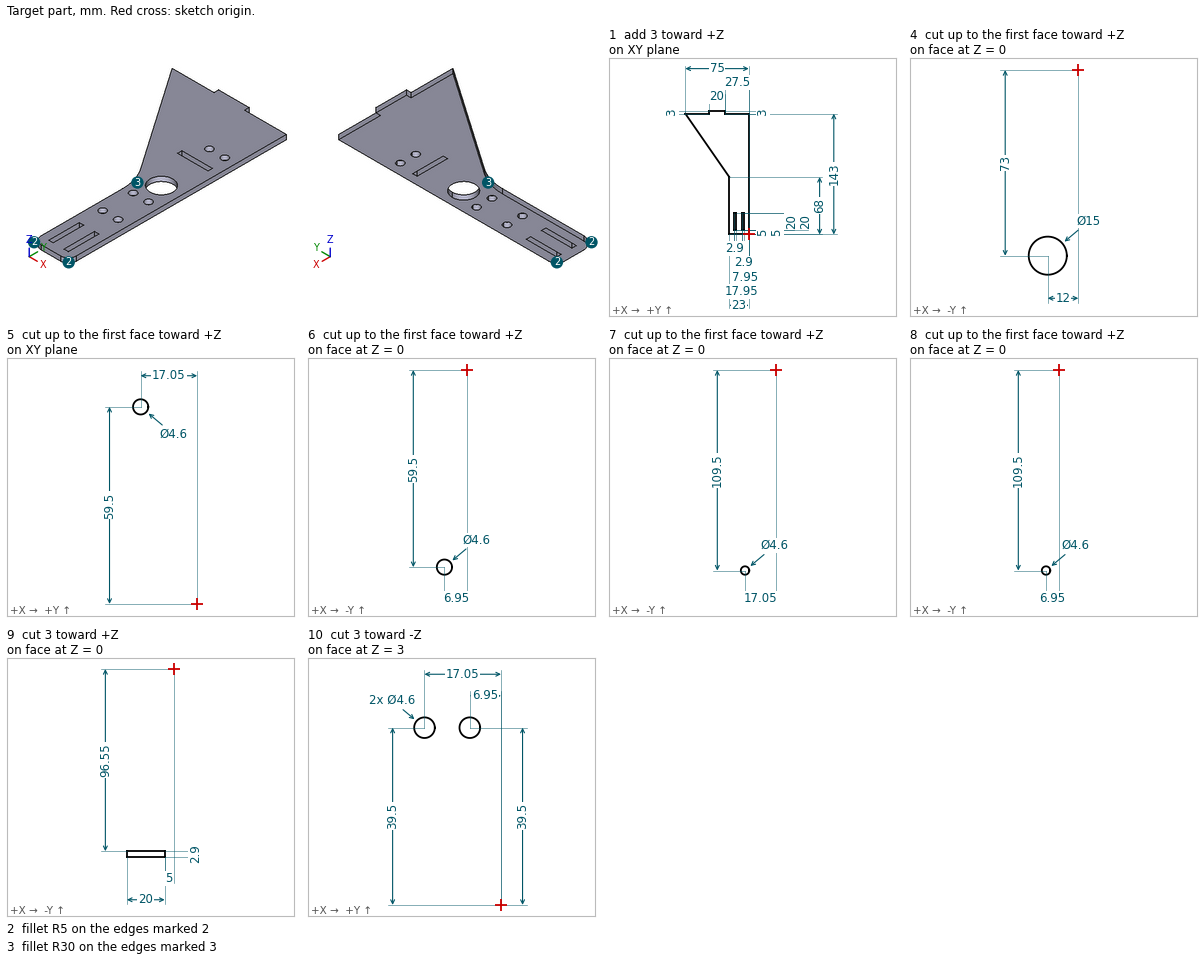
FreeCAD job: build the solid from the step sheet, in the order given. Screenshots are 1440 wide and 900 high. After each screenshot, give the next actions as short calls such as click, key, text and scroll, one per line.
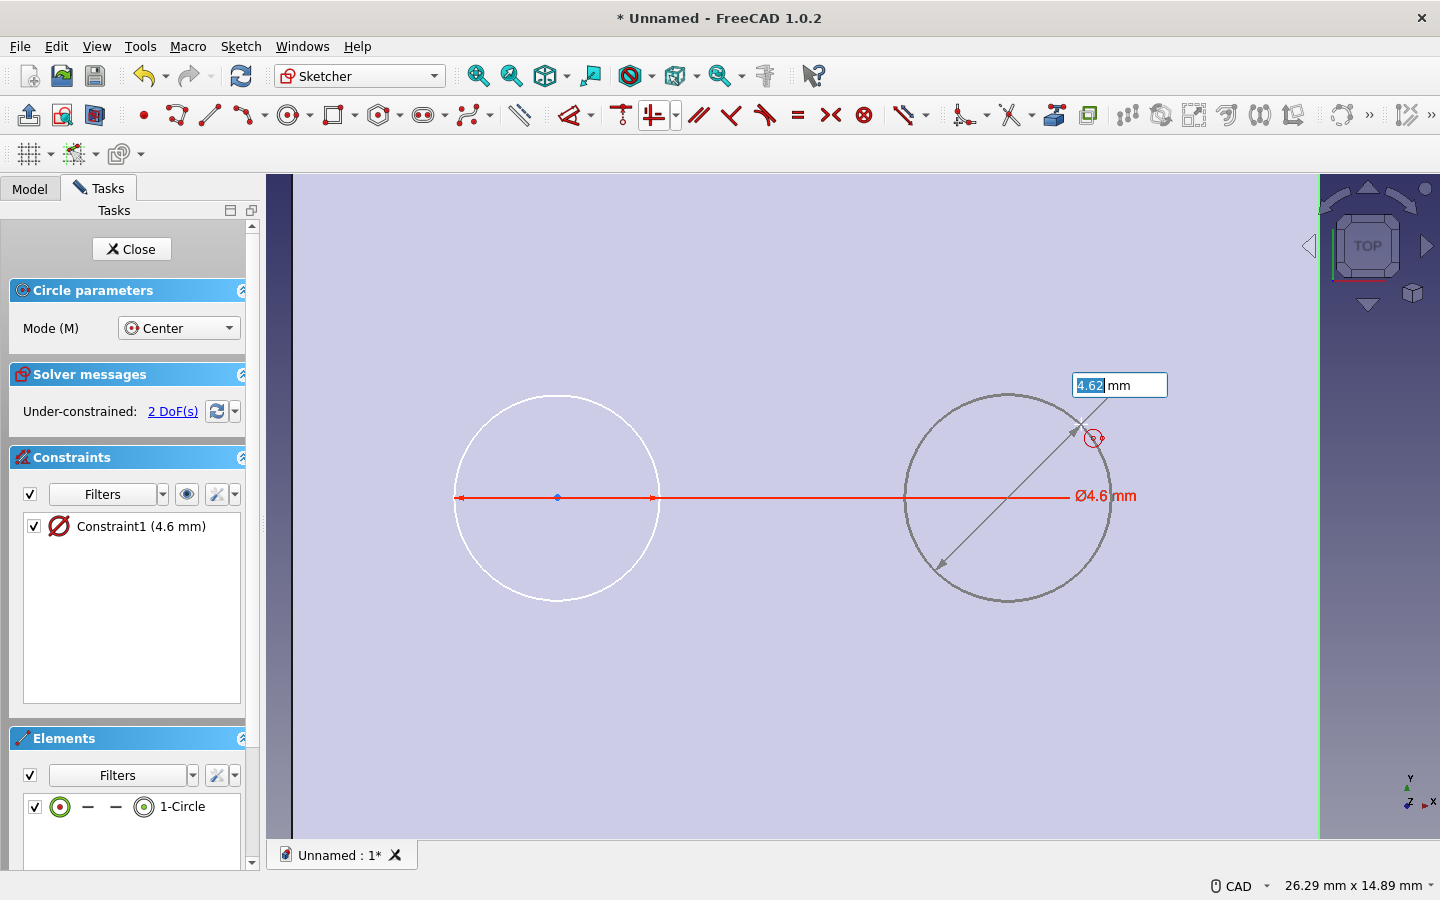
text(4.6)
key(Return)
key(Escape)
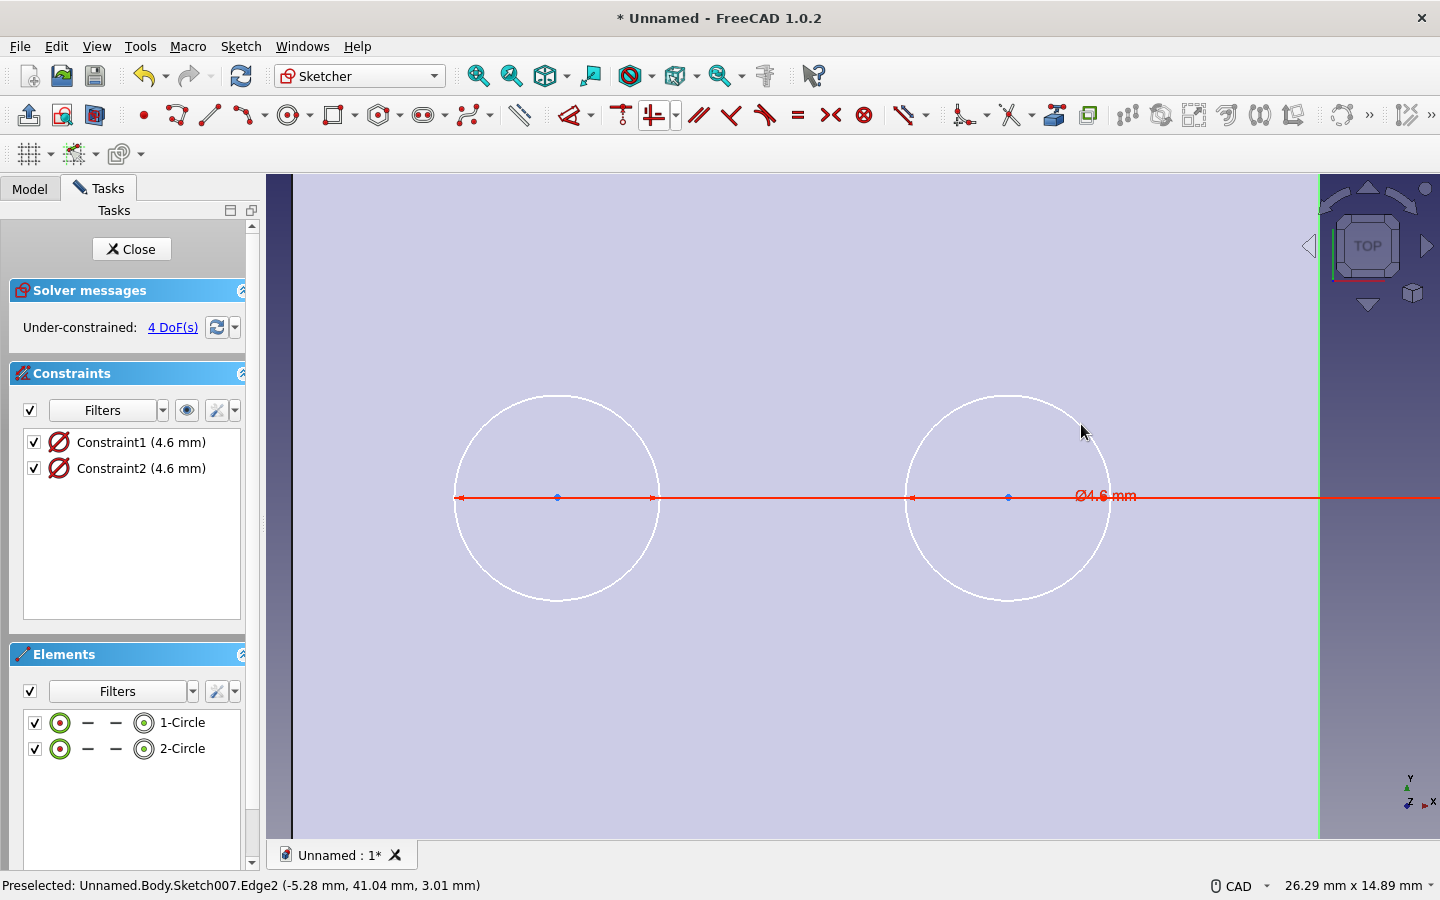
key(d)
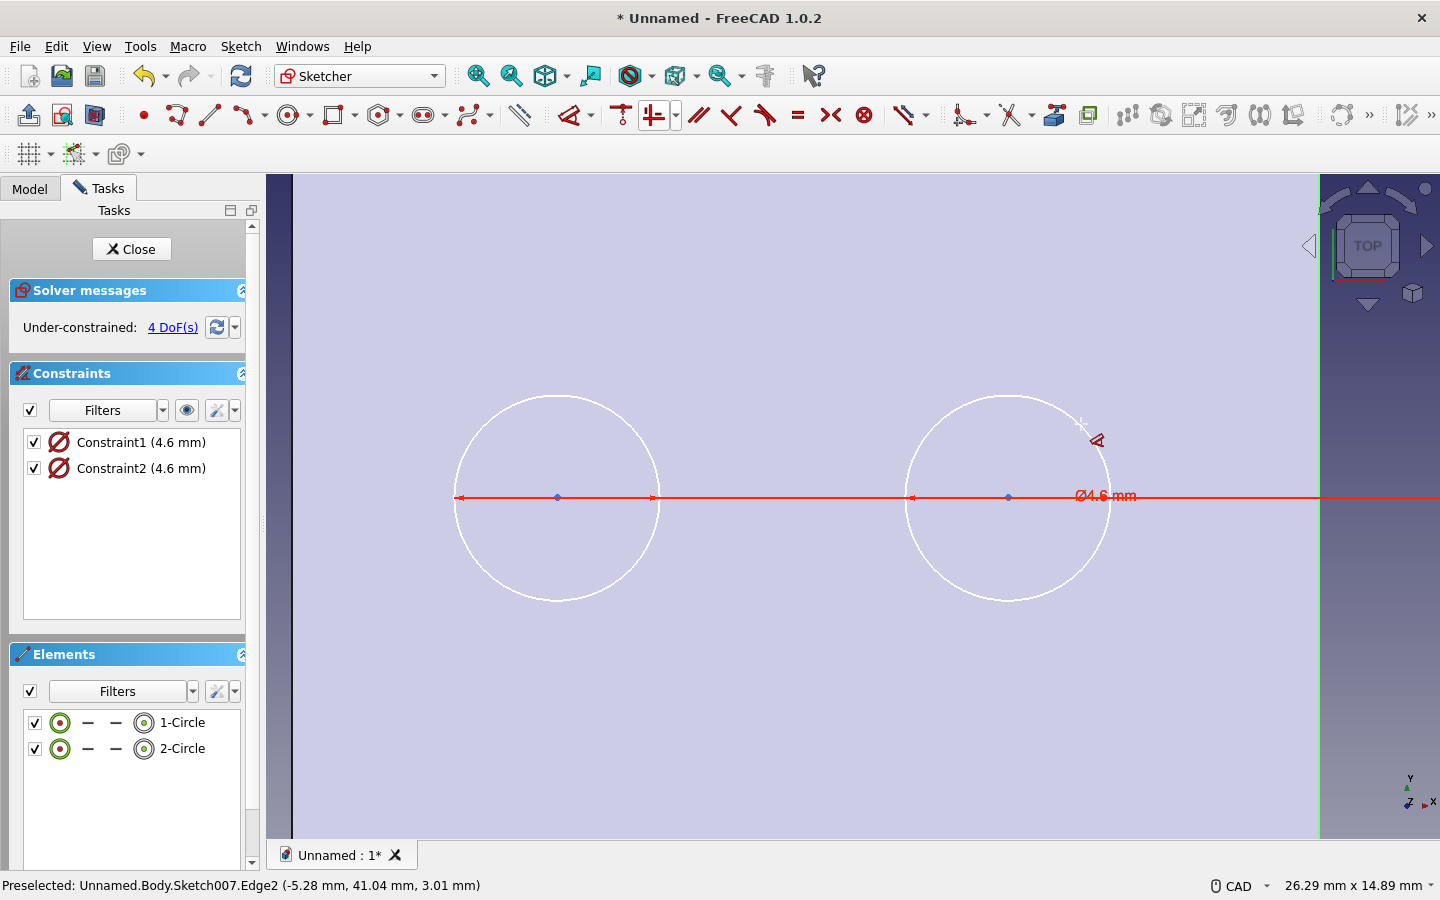
click(557, 498)
click(523, 655)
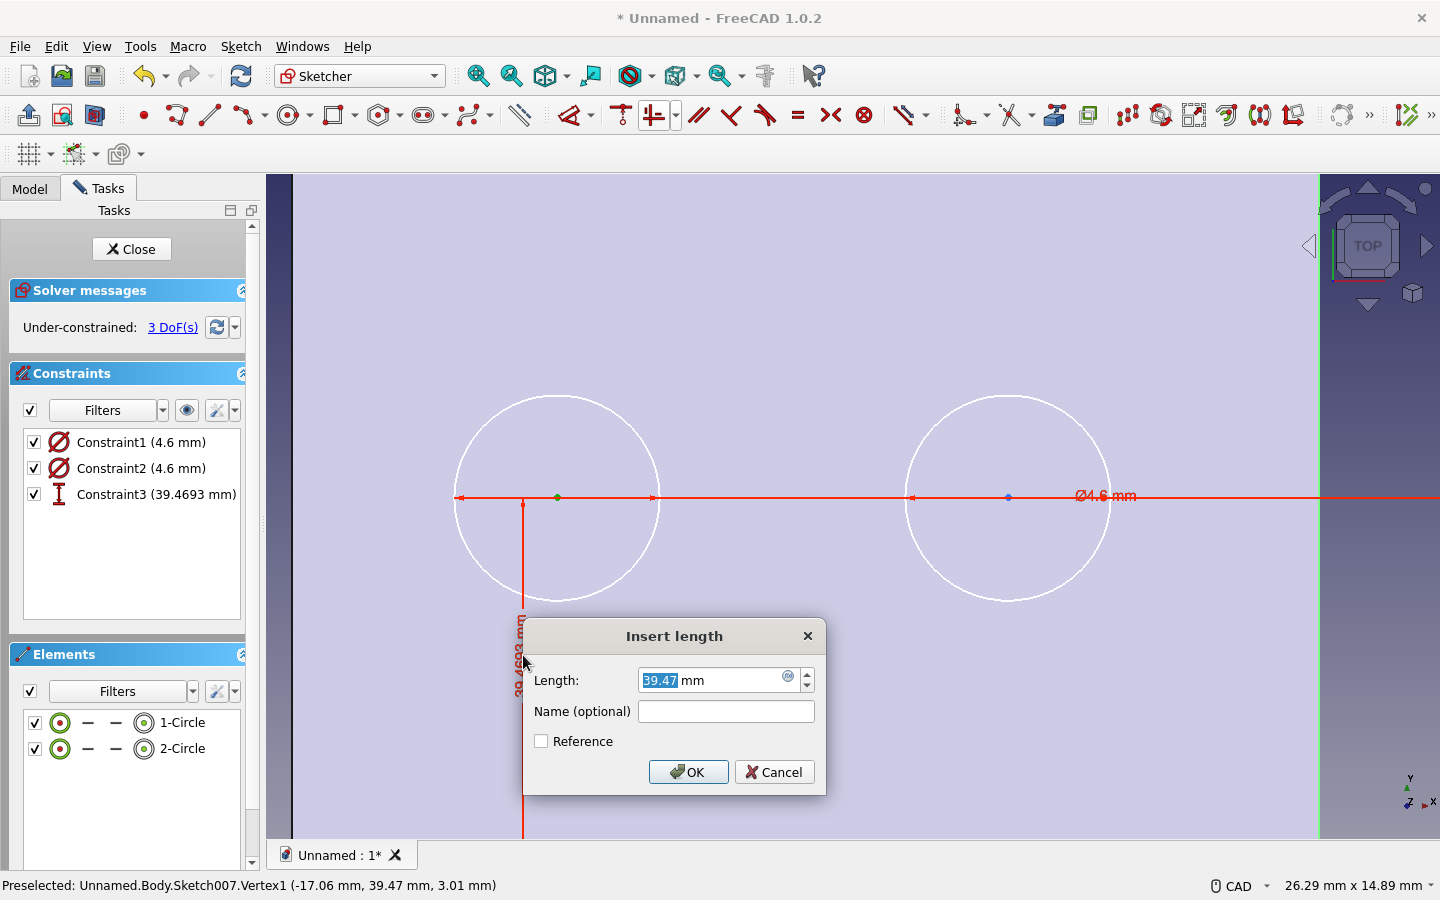
text(39.5)
key(Return)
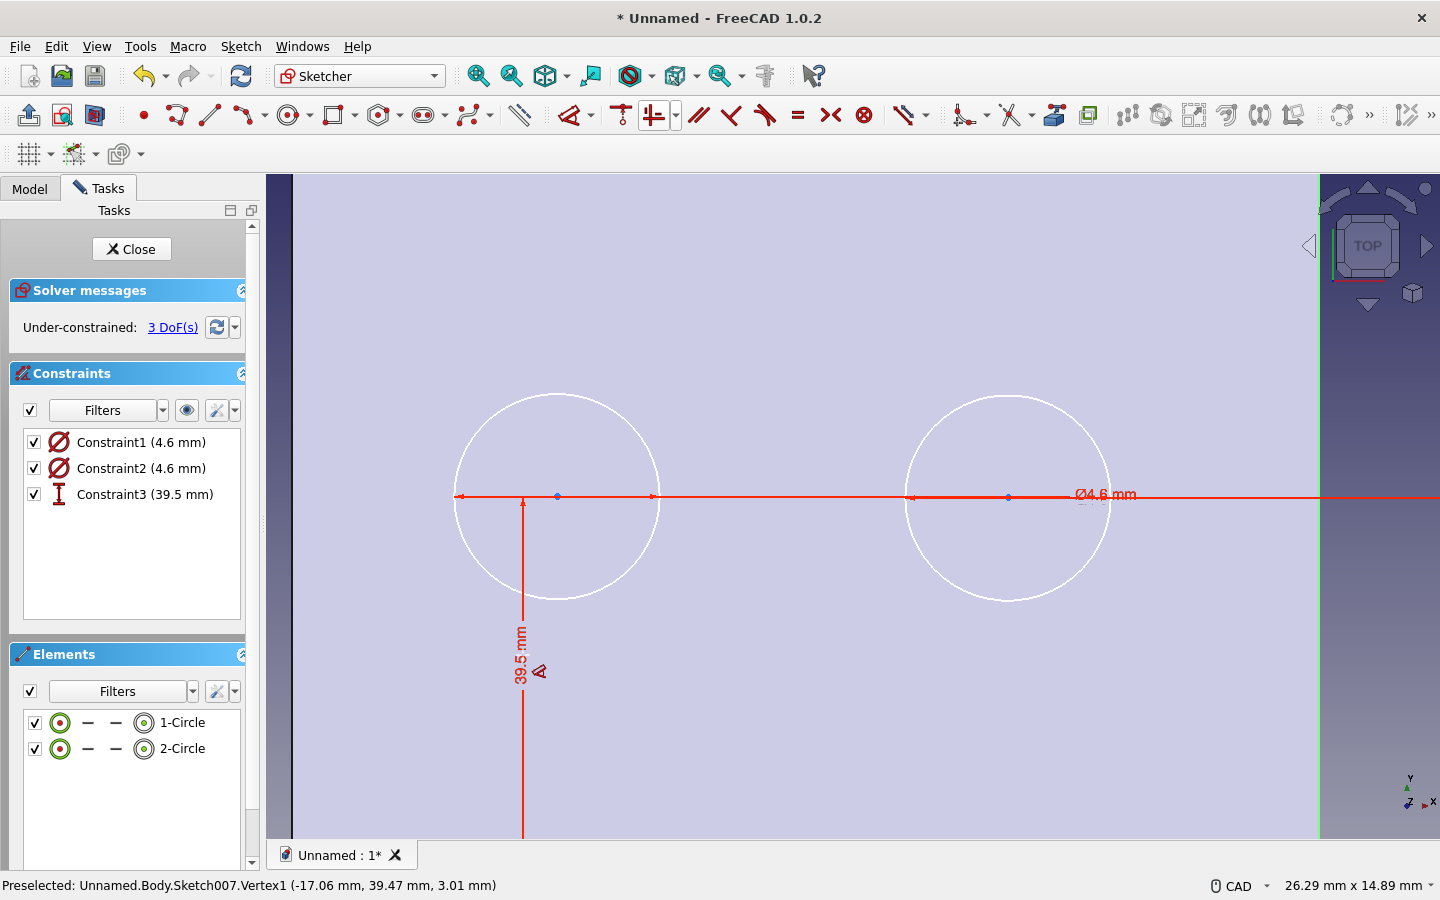
click(1008, 498)
click(1142, 464)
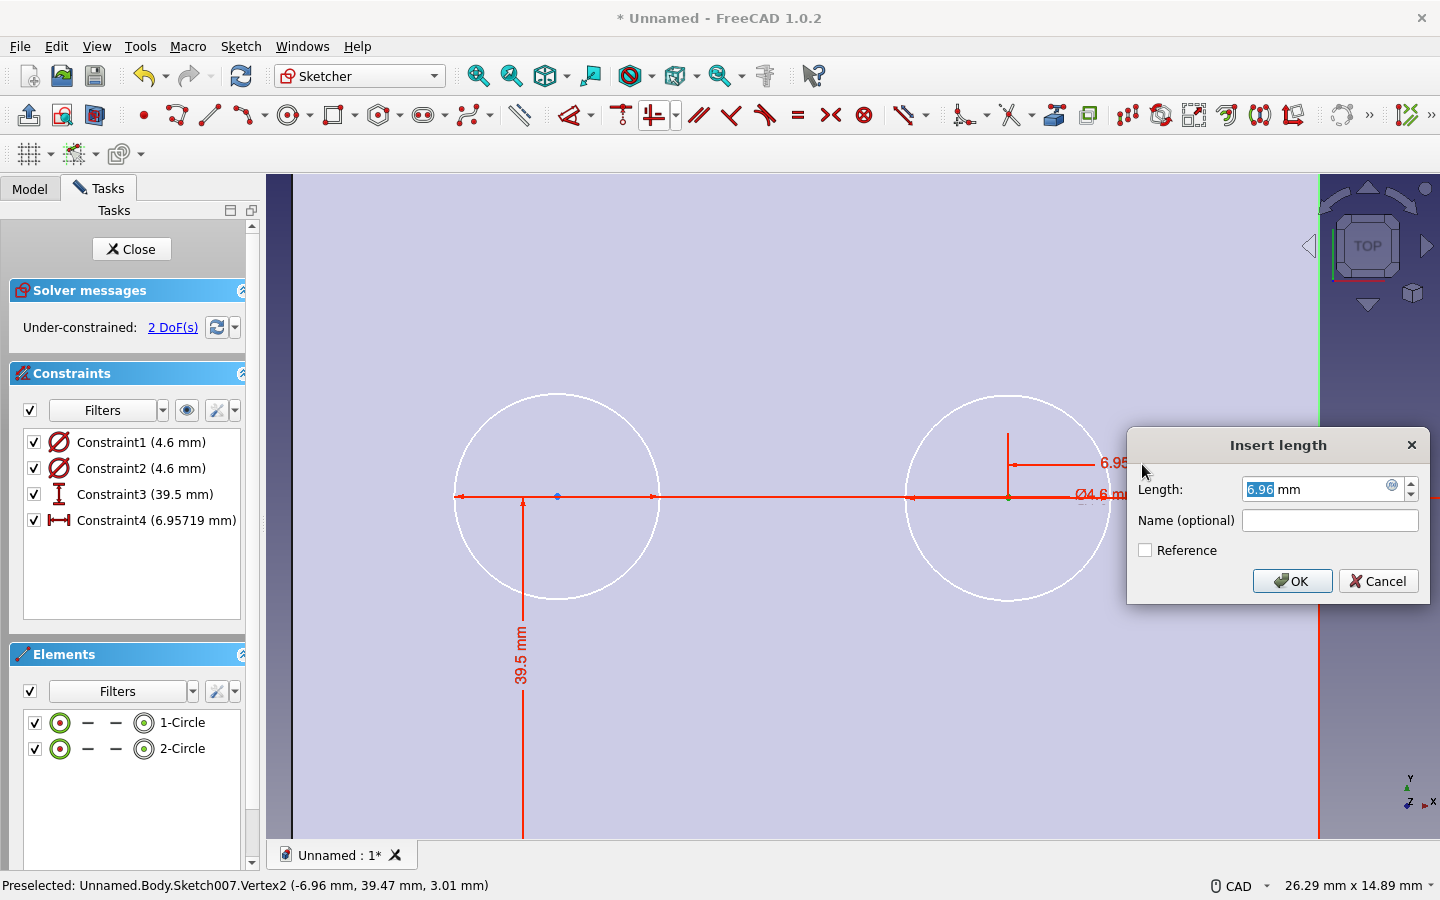
text(6.95)
key(Return)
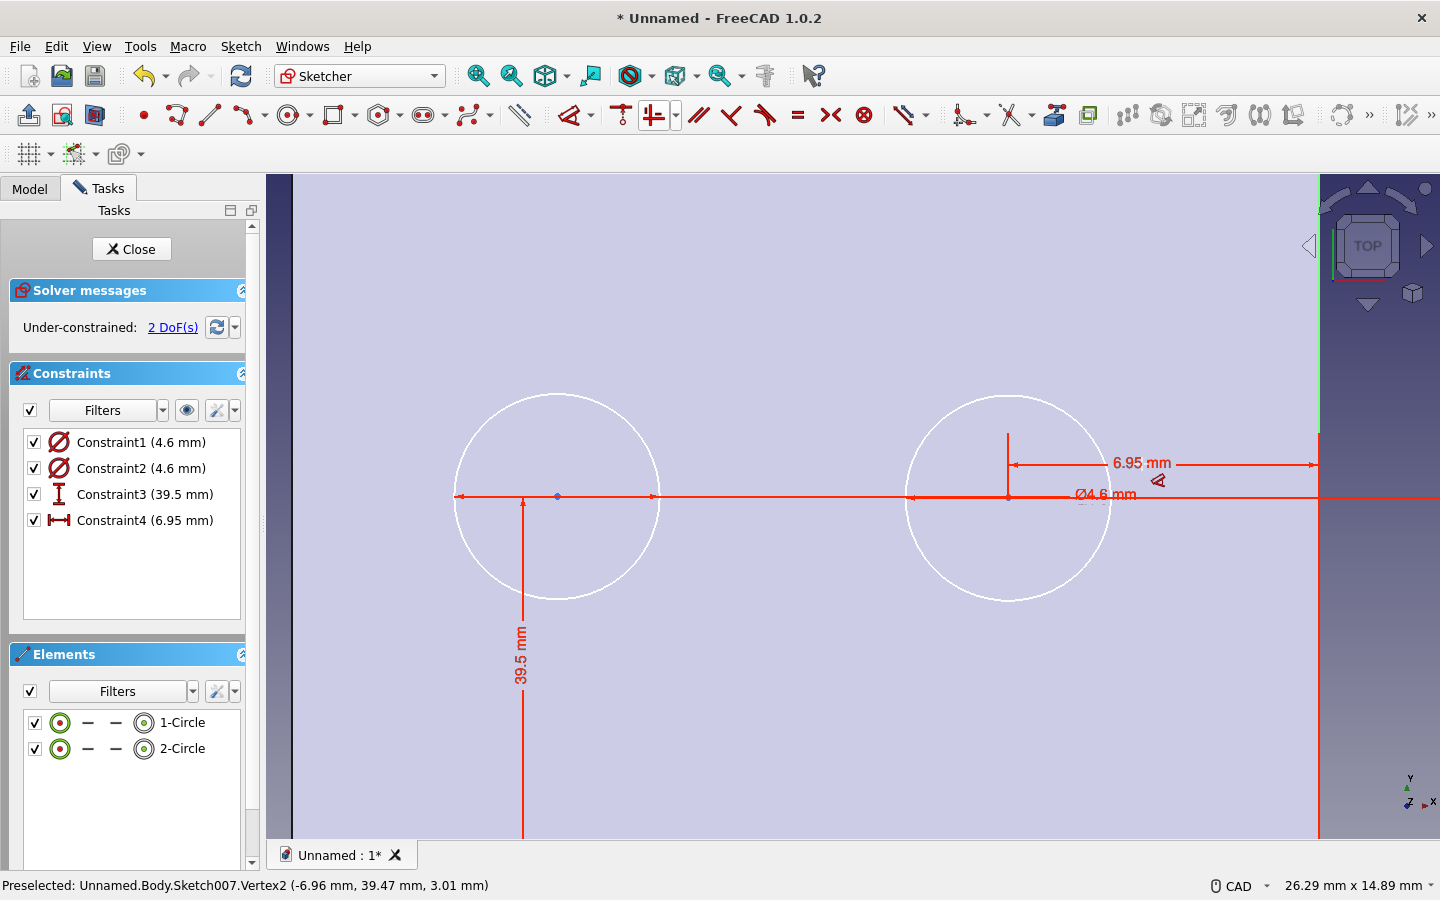
click(1008, 498)
click(974, 655)